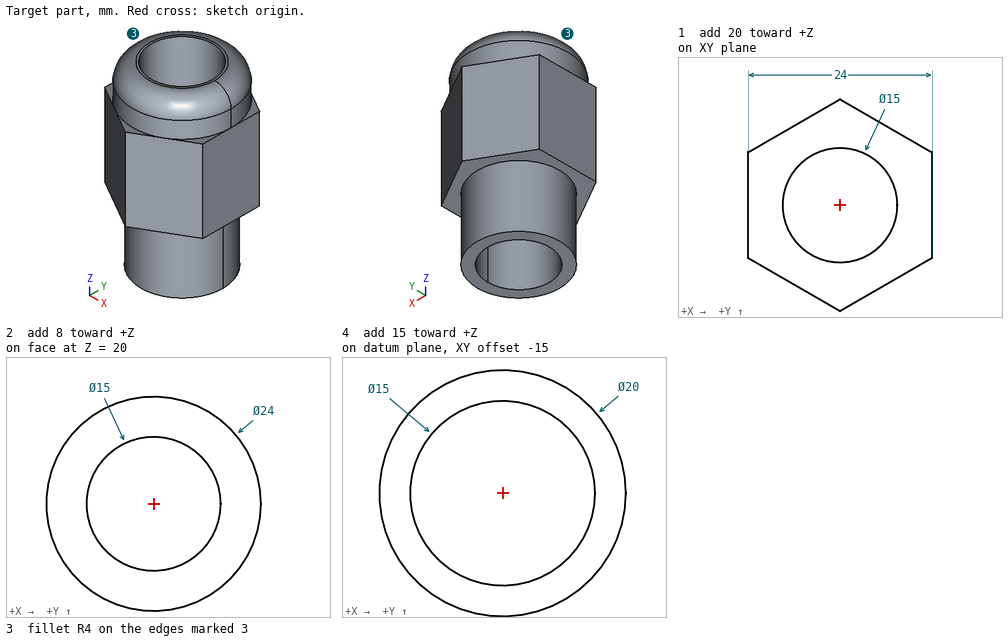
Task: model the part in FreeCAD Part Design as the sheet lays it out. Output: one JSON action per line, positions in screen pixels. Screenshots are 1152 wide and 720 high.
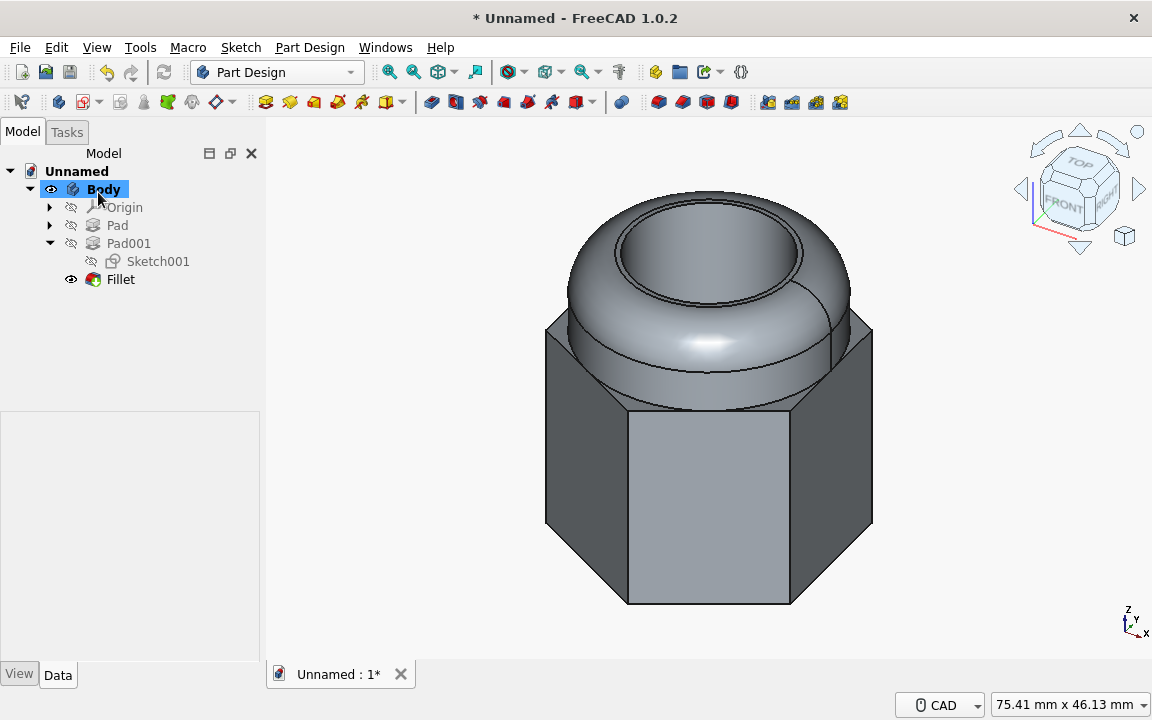
{"action": "left_click", "coordinate": [50, 207]}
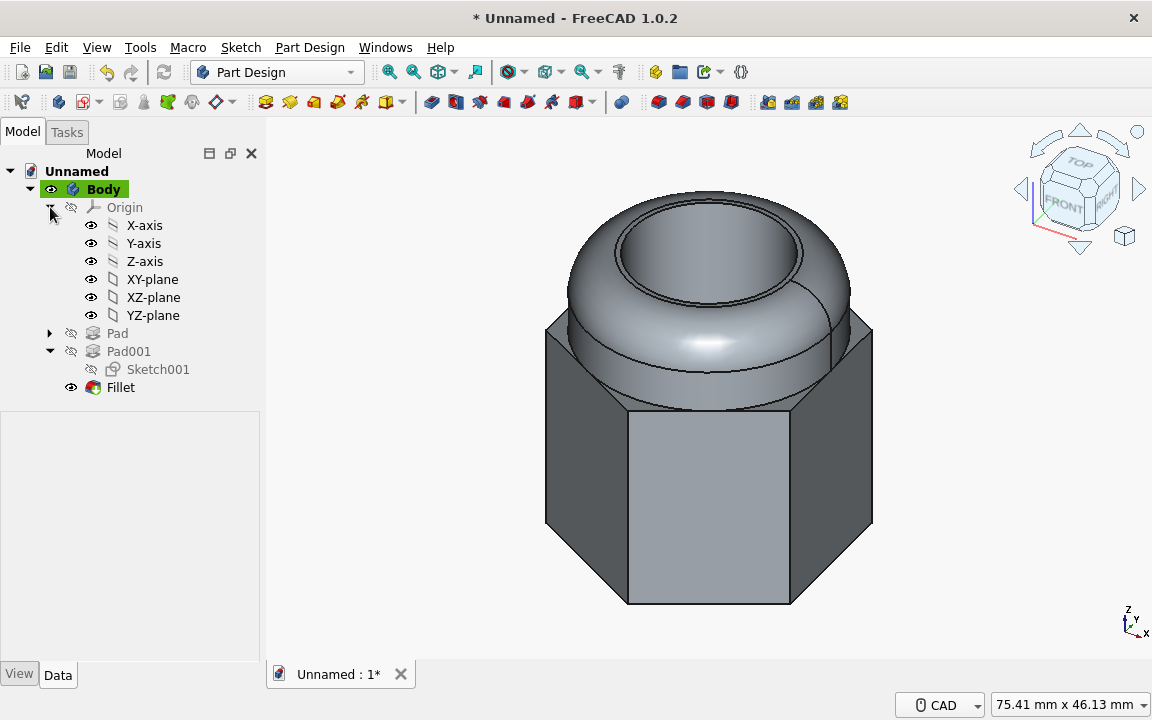
{"action": "left_click", "coordinate": [136, 279]}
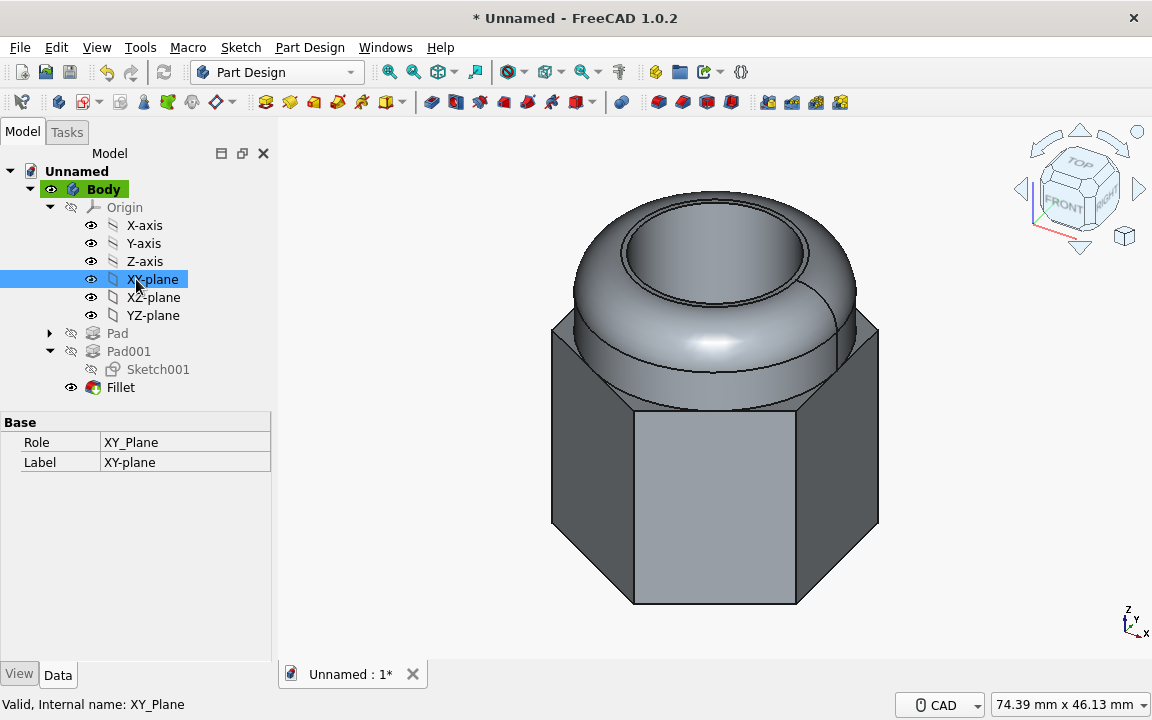
{"action": "left_click", "coordinate": [216, 102]}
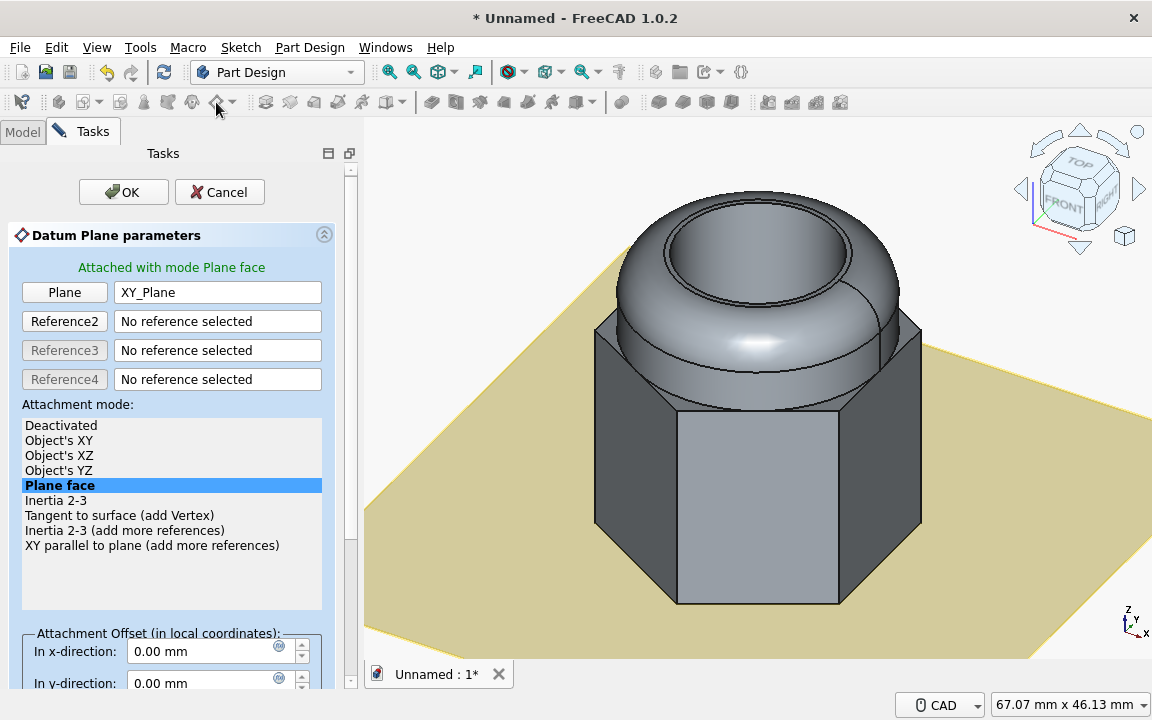
{"action": "scroll", "coordinate": [351, 426], "scroll_direction": "down", "scroll_amount": 2}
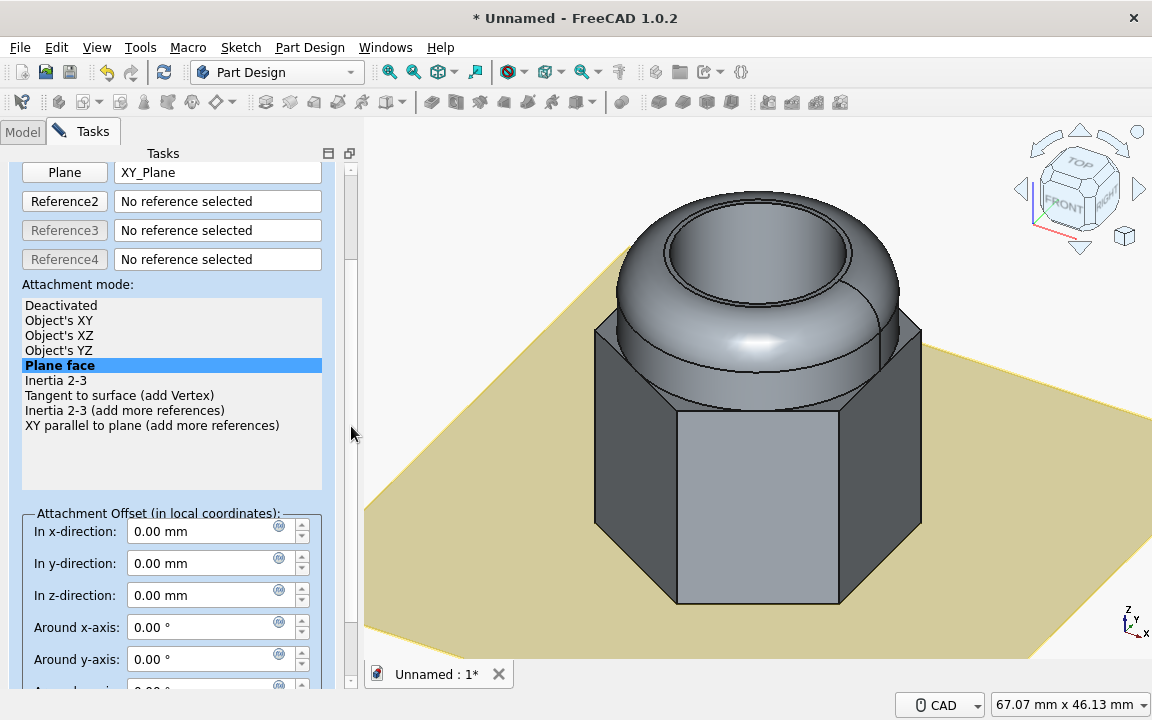
{"action": "triple_click", "coordinate": [210, 595]}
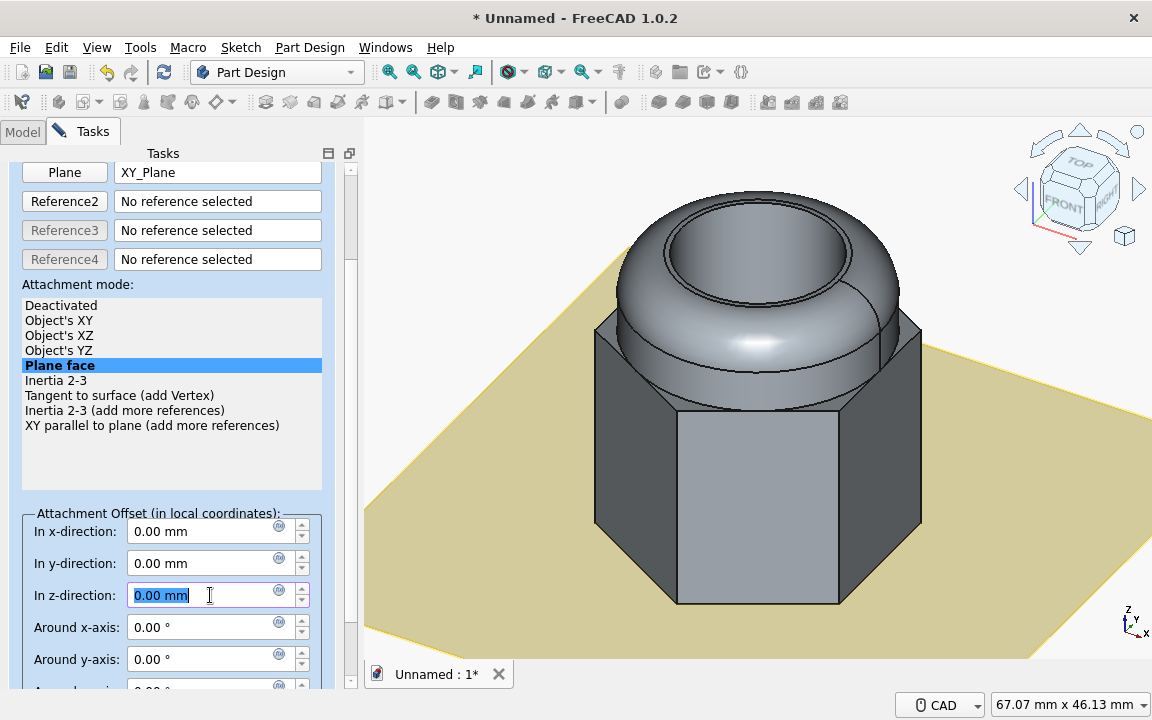
{"action": "type", "text": "-15"}
{"action": "key", "text": "Tab"}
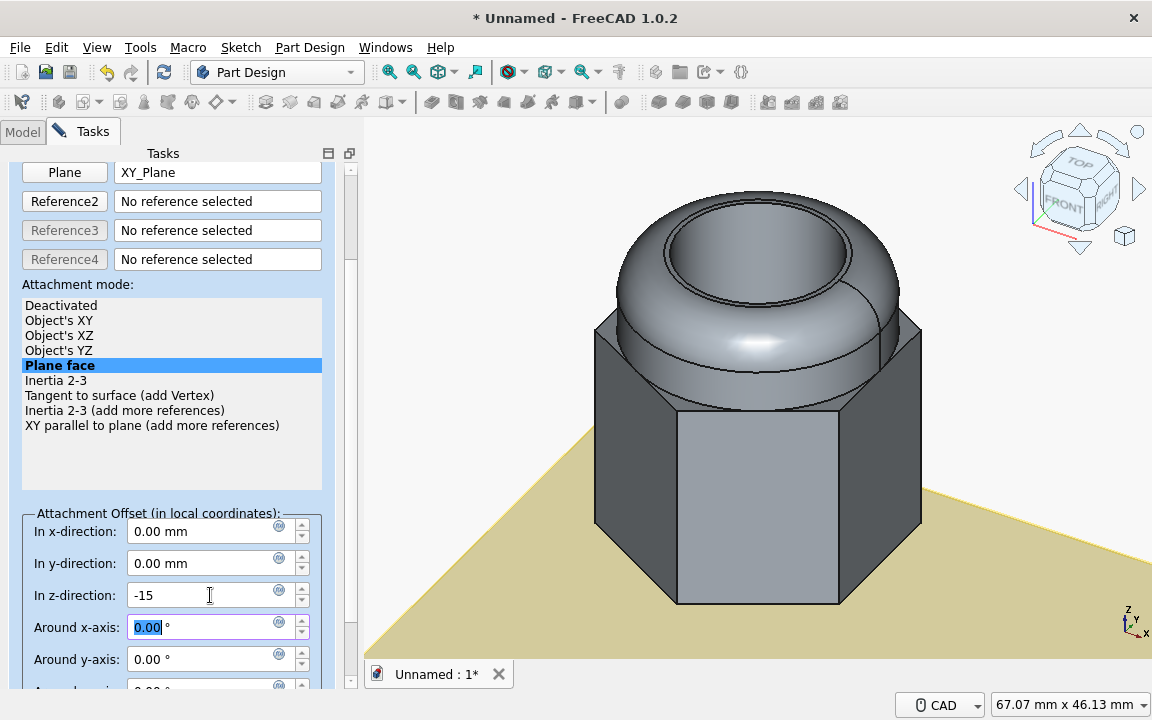
{"action": "scroll", "coordinate": [351, 426], "scroll_direction": "up", "scroll_amount": 3}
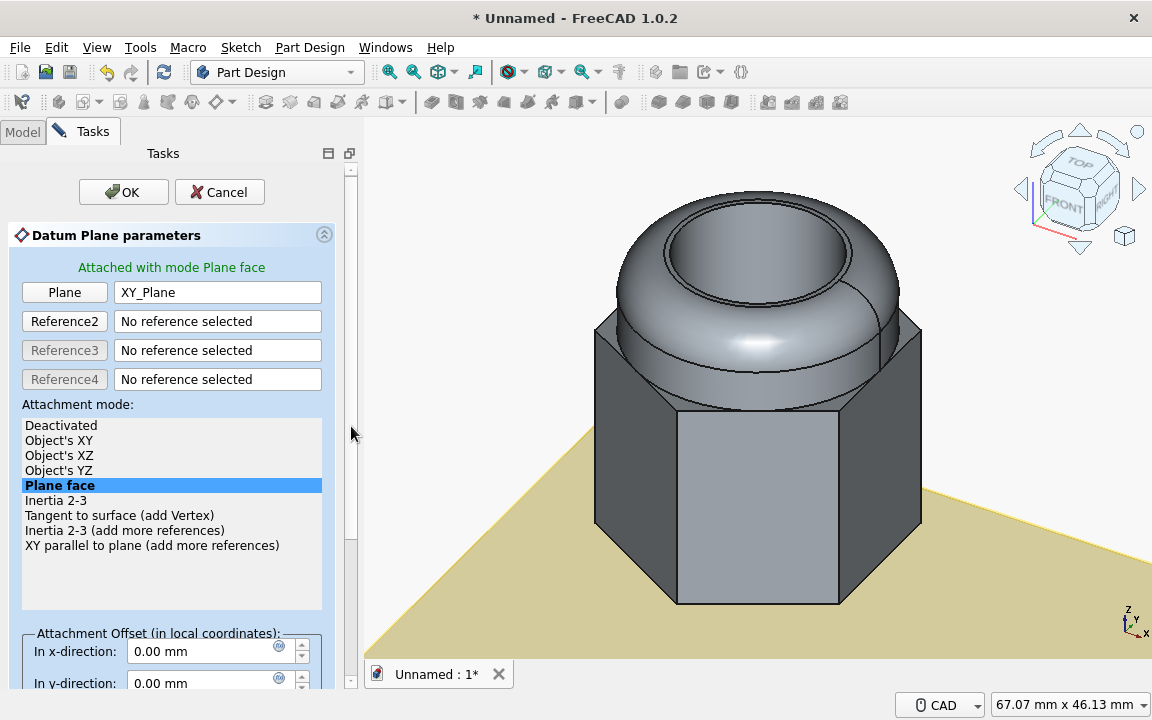
{"action": "left_click", "coordinate": [124, 192]}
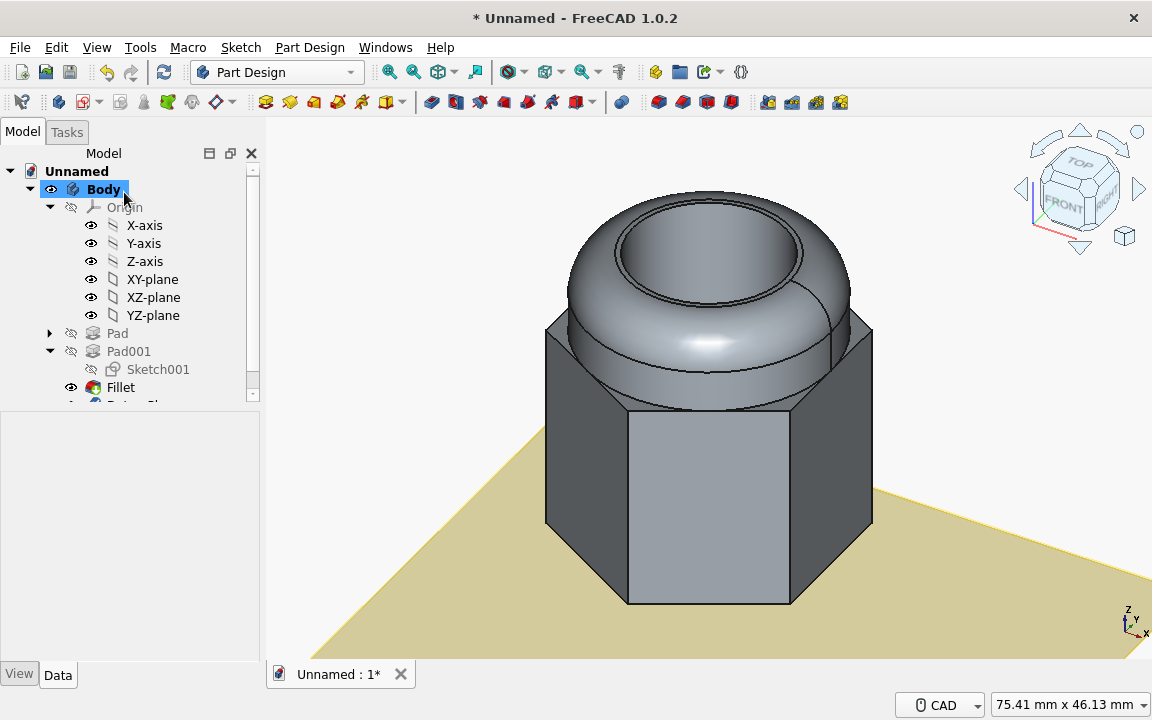
{"action": "scroll", "coordinate": [100, 275], "scroll_direction": "down", "scroll_amount": 3}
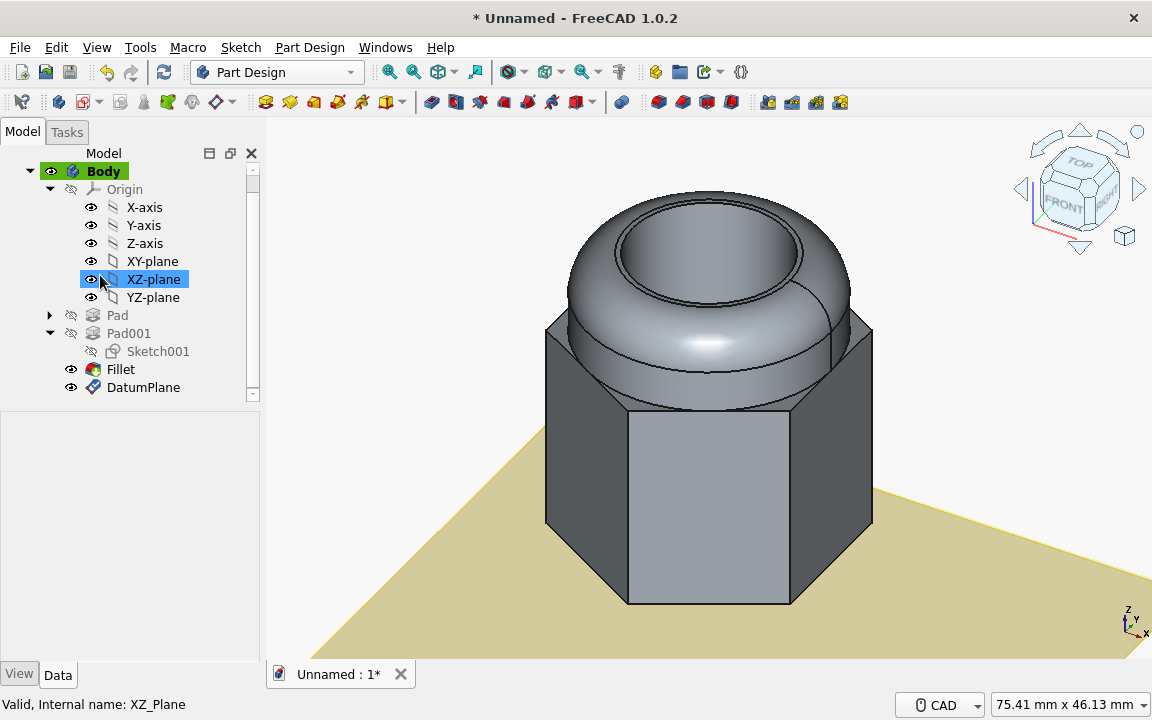
{"action": "left_click", "coordinate": [116, 387]}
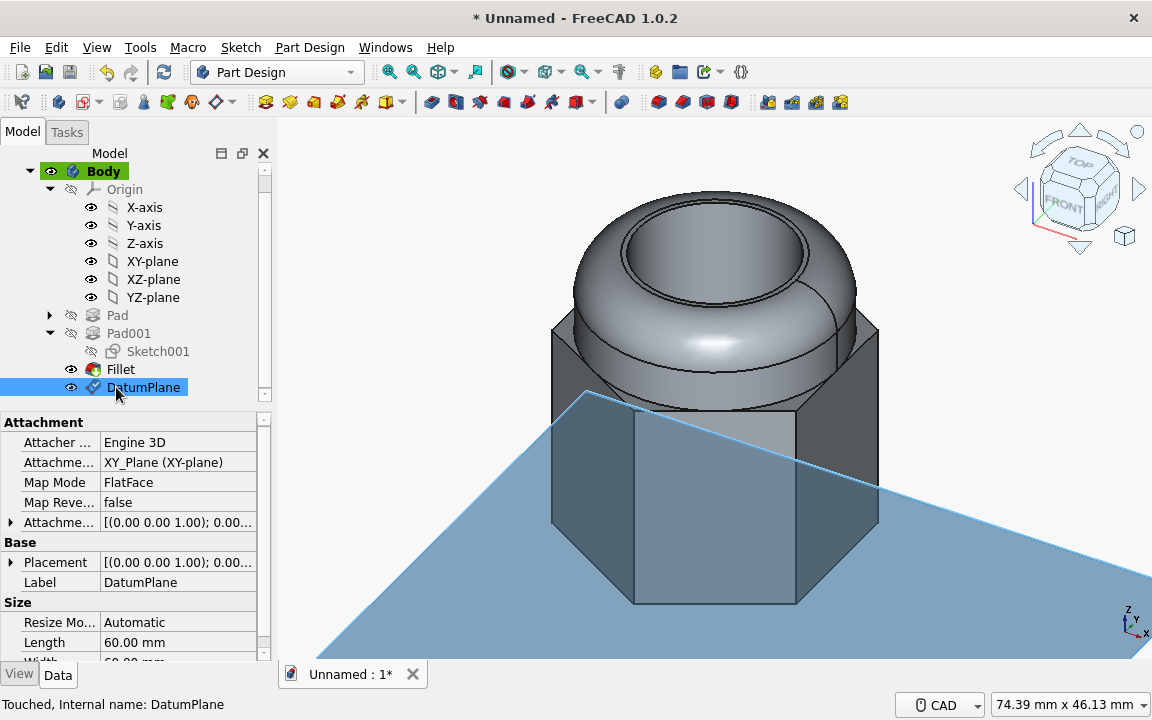
{"action": "left_click", "coordinate": [84, 102]}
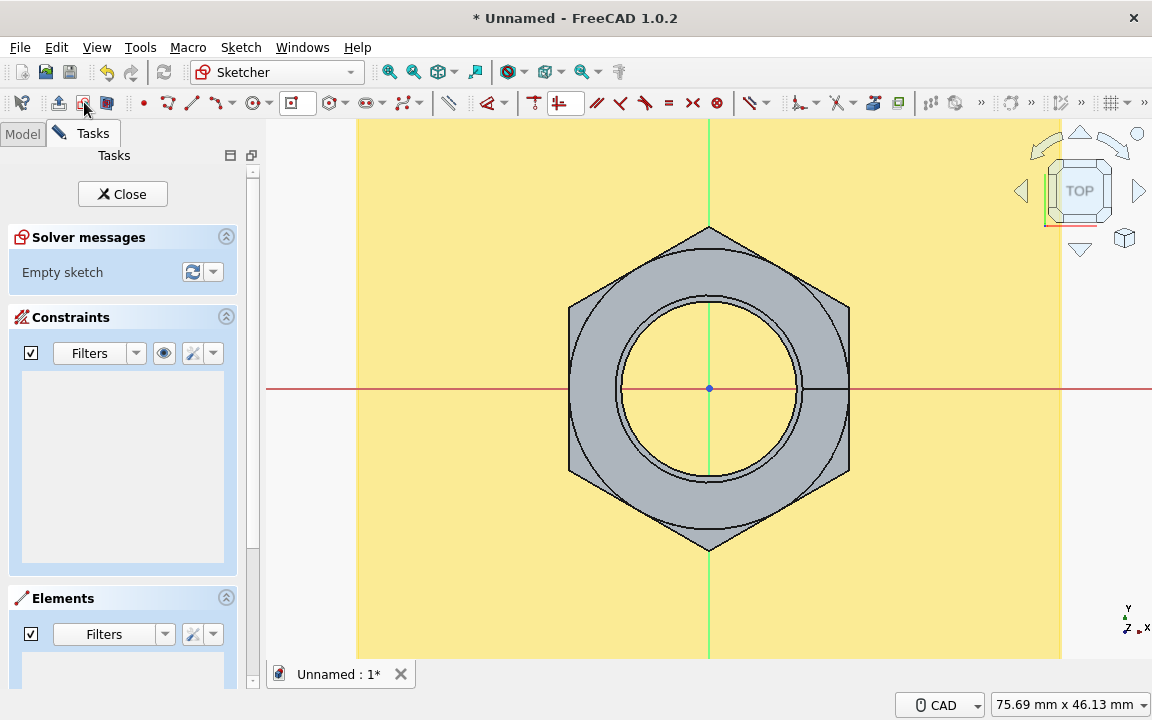
{"action": "key", "text": "q s"}